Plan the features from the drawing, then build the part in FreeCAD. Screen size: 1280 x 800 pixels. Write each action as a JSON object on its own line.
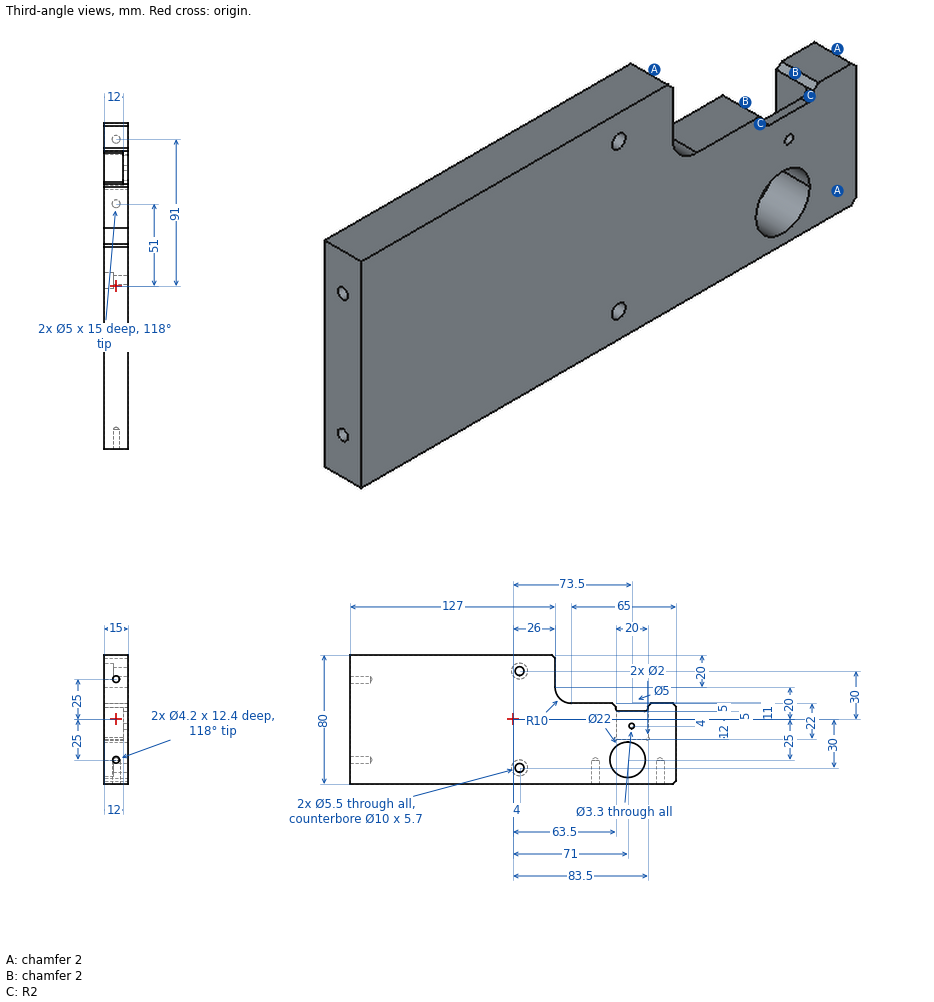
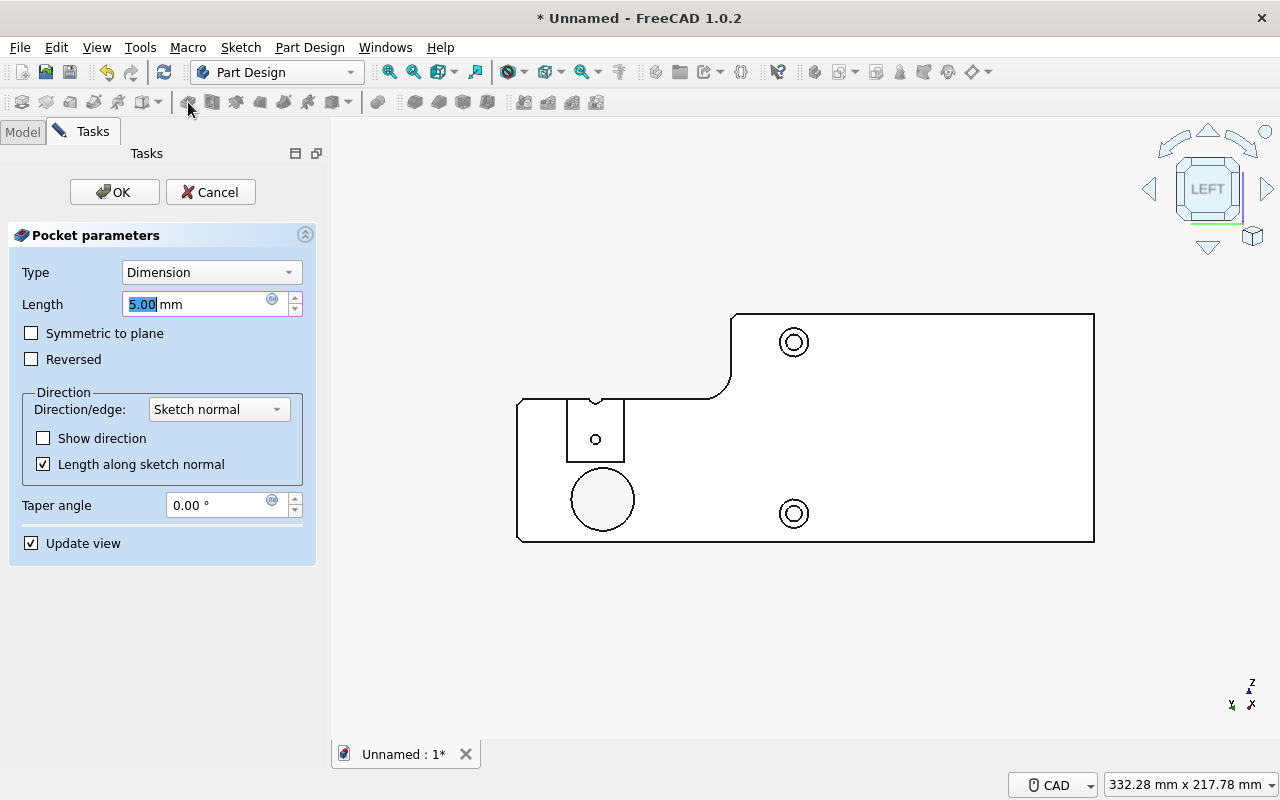
{"action": "type", "text": "12"}
{"action": "key", "text": "Tab"}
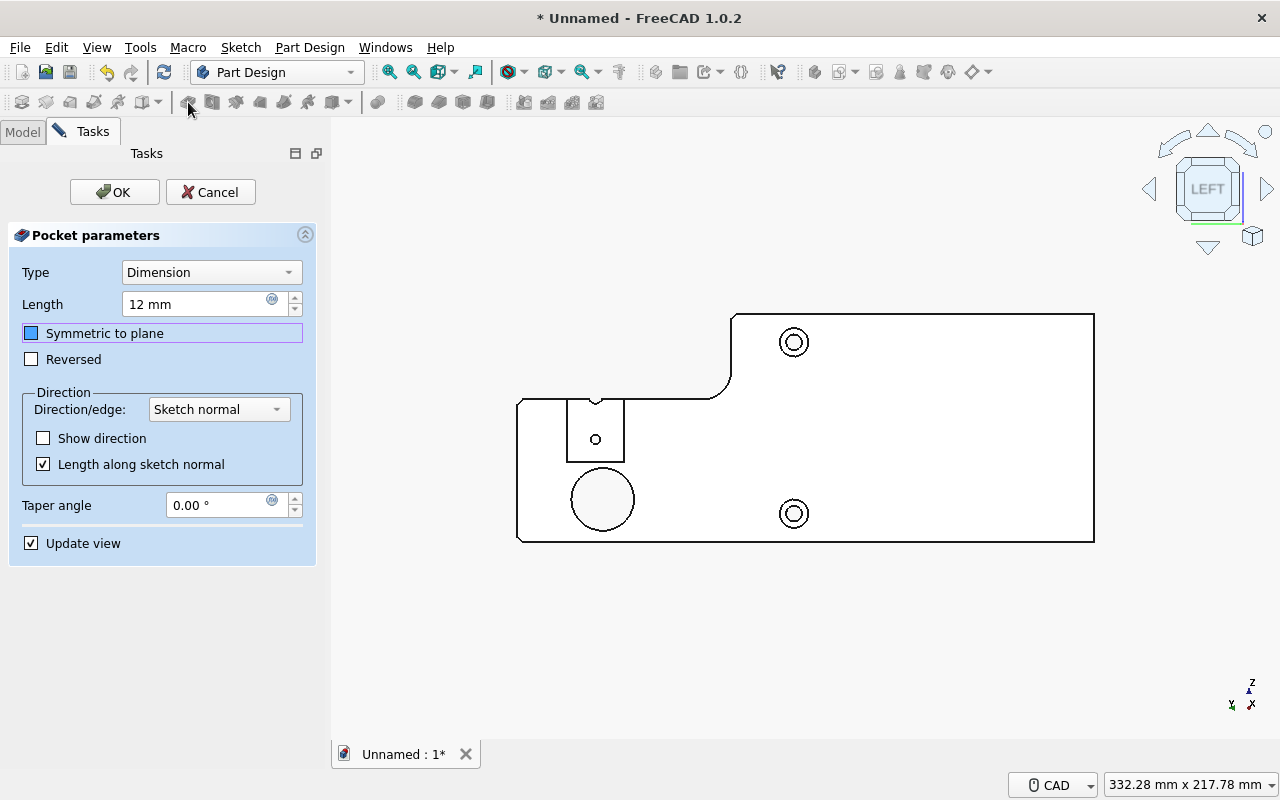
{"action": "left_click", "coordinate": [115, 192]}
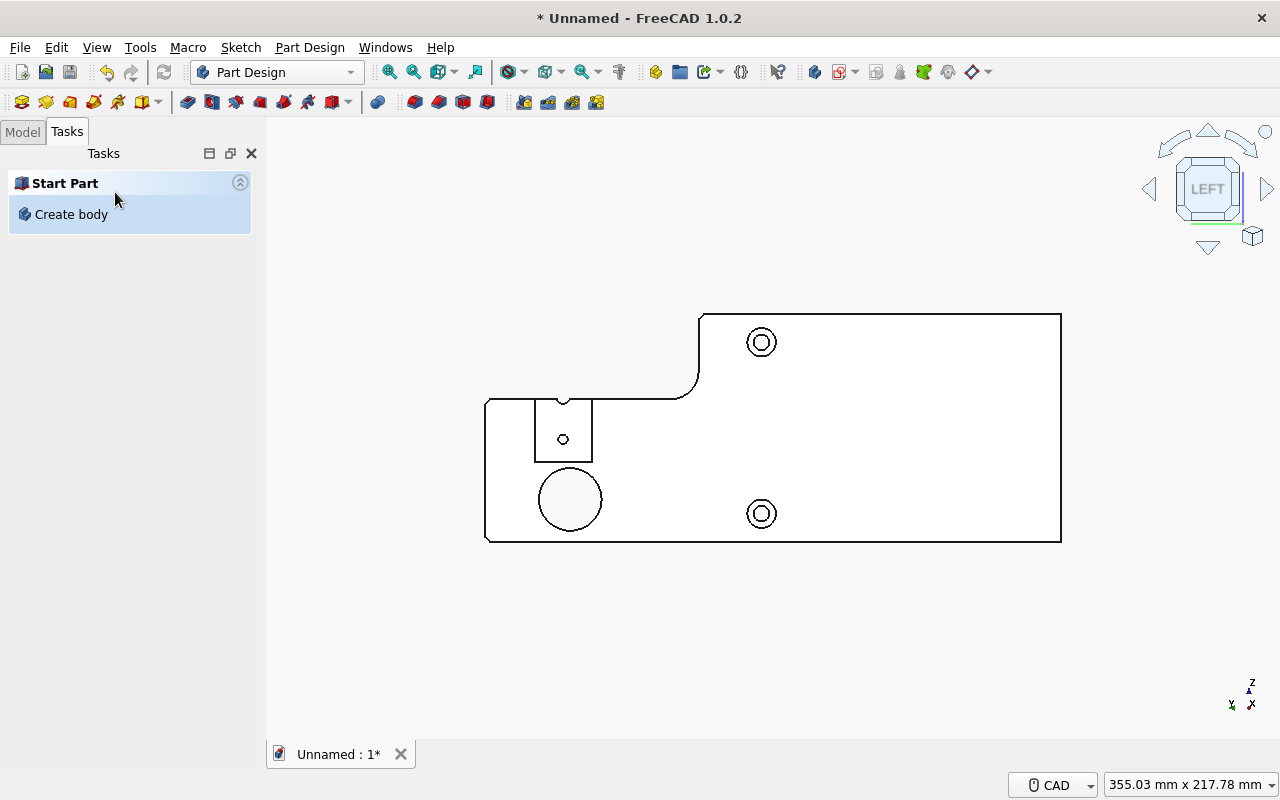
{"action": "left_click", "coordinate": [571, 421]}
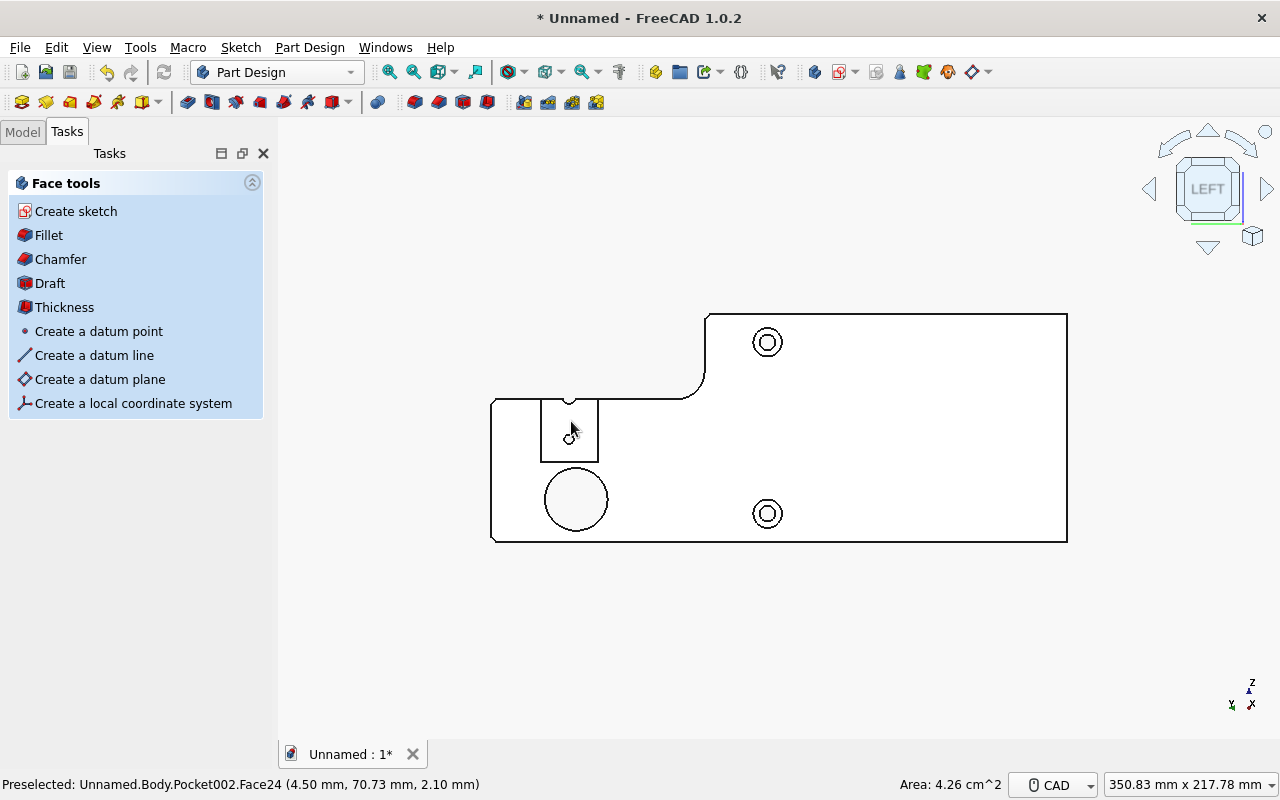
{"action": "left_click", "coordinate": [840, 72]}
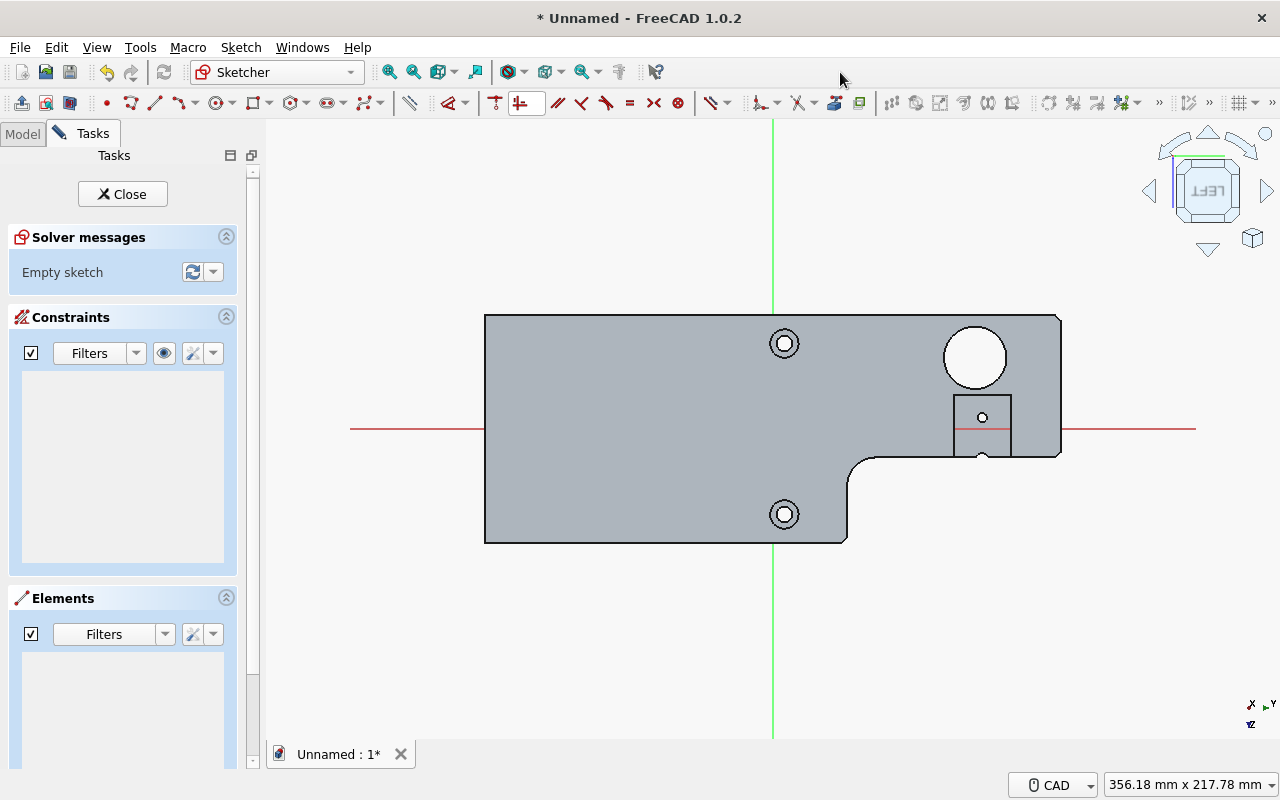
{"action": "left_click", "coordinate": [70, 104]}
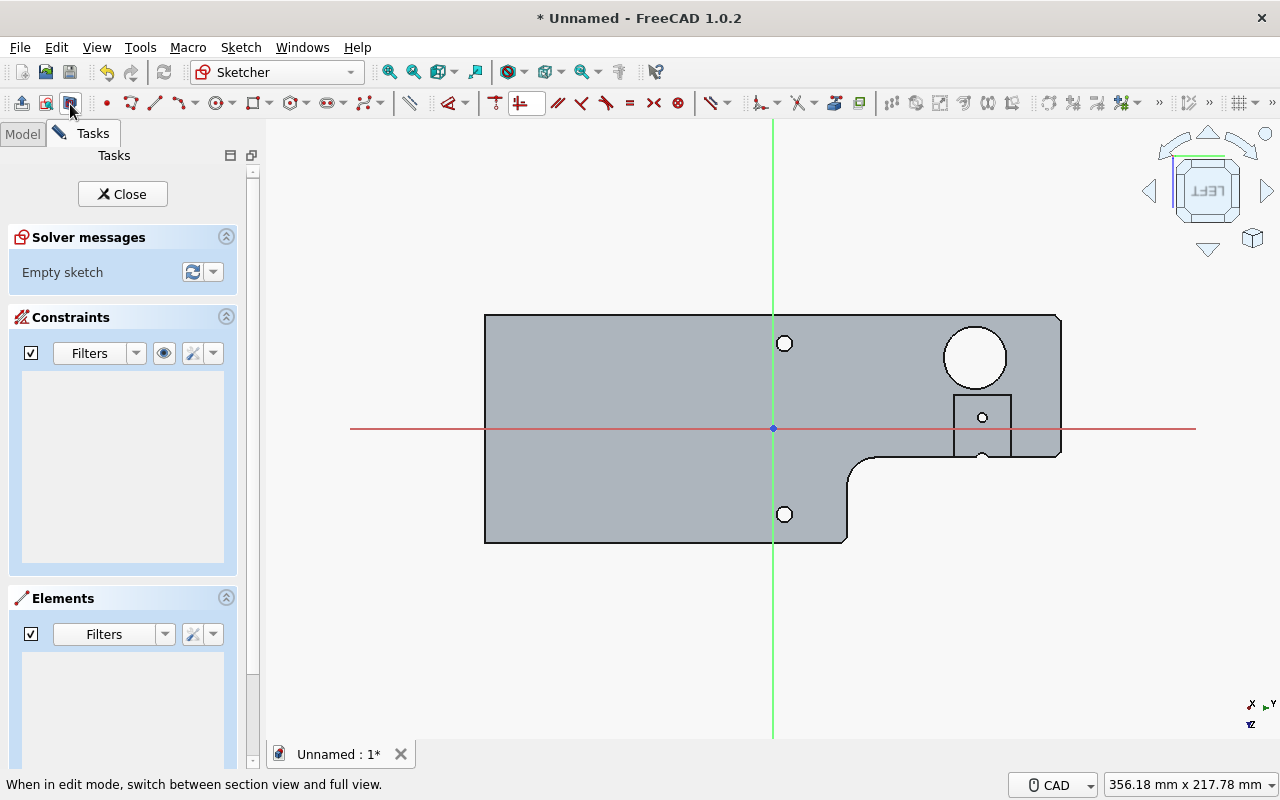
{"action": "scroll", "coordinate": [1010, 452], "scroll_direction": "up", "scroll_amount": 12}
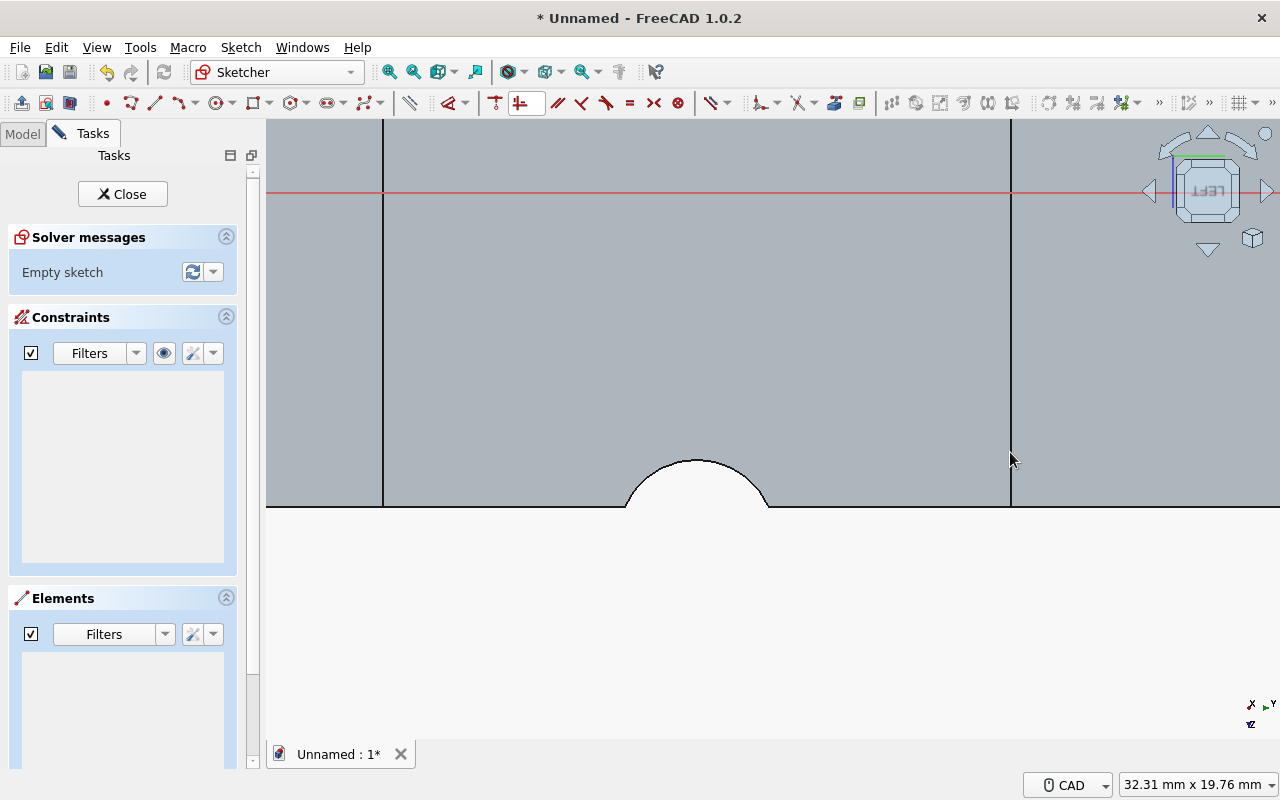
{"action": "left_click", "coordinate": [254, 104]}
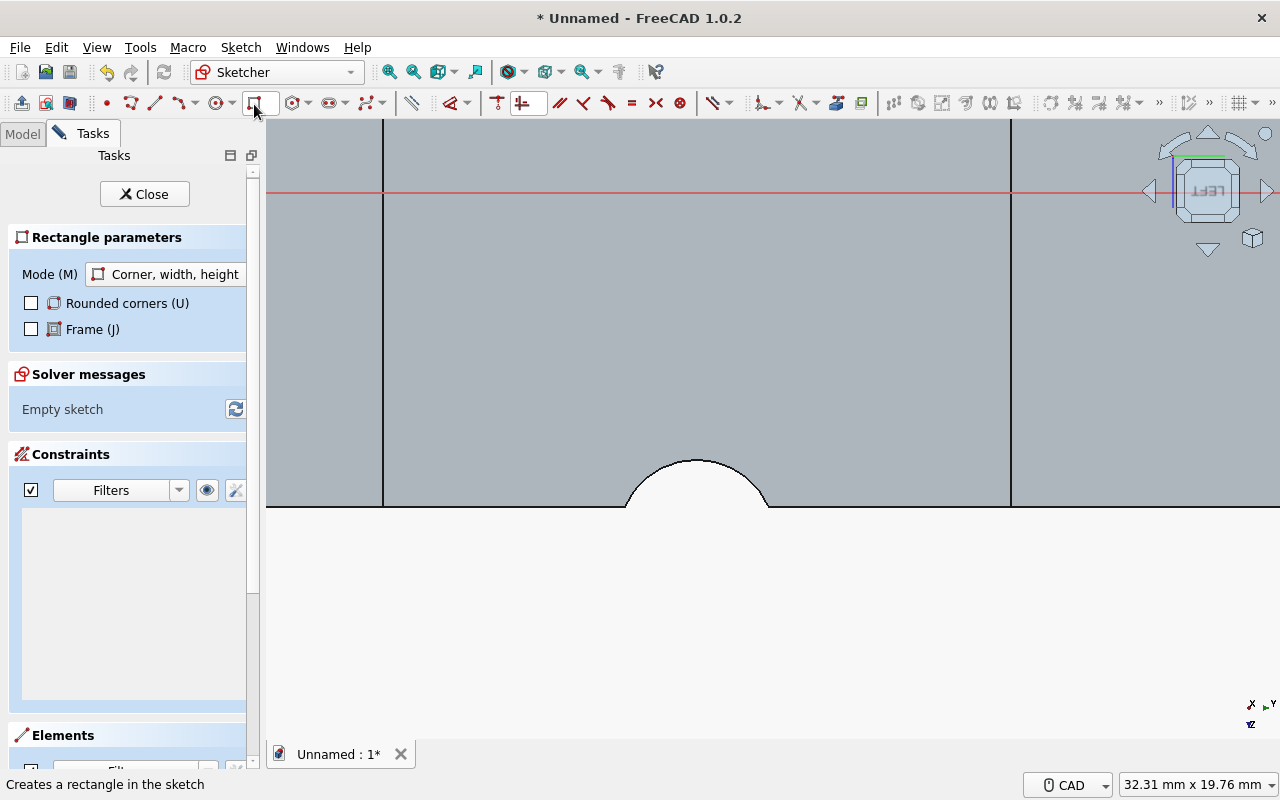
{"action": "left_click", "coordinate": [383, 350]}
{"action": "left_click", "coordinate": [1011, 507]}
{"action": "key", "text": "Escape"}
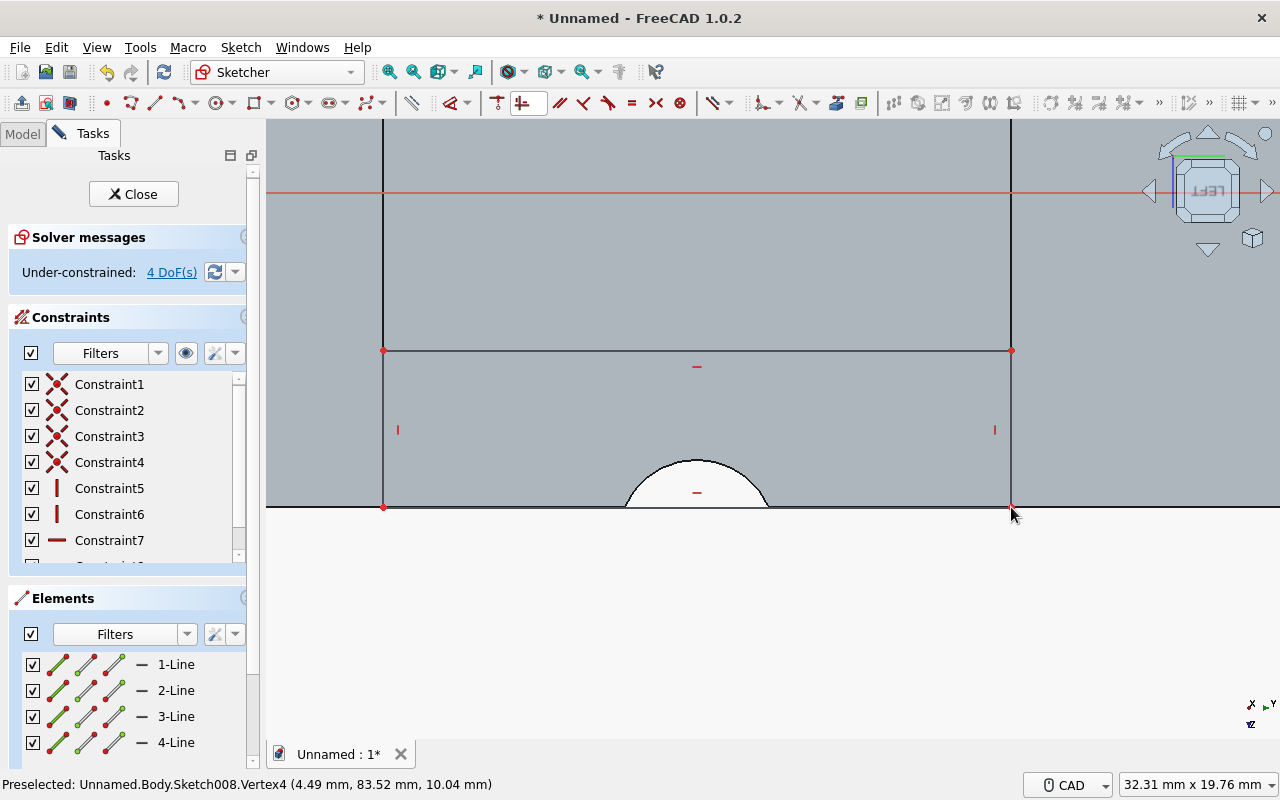
{"action": "left_click", "coordinate": [450, 104]}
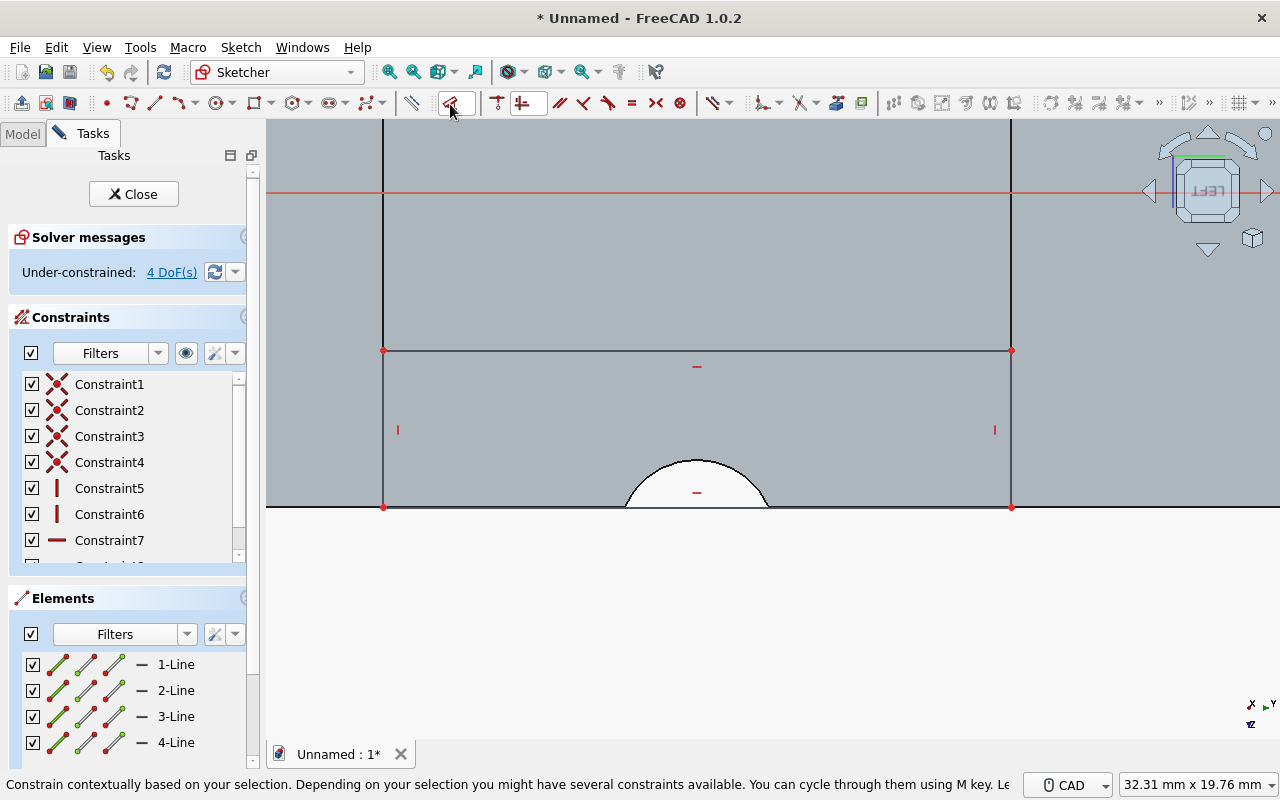
{"action": "left_click", "coordinate": [383, 398]}
{"action": "left_click", "coordinate": [349, 429]}